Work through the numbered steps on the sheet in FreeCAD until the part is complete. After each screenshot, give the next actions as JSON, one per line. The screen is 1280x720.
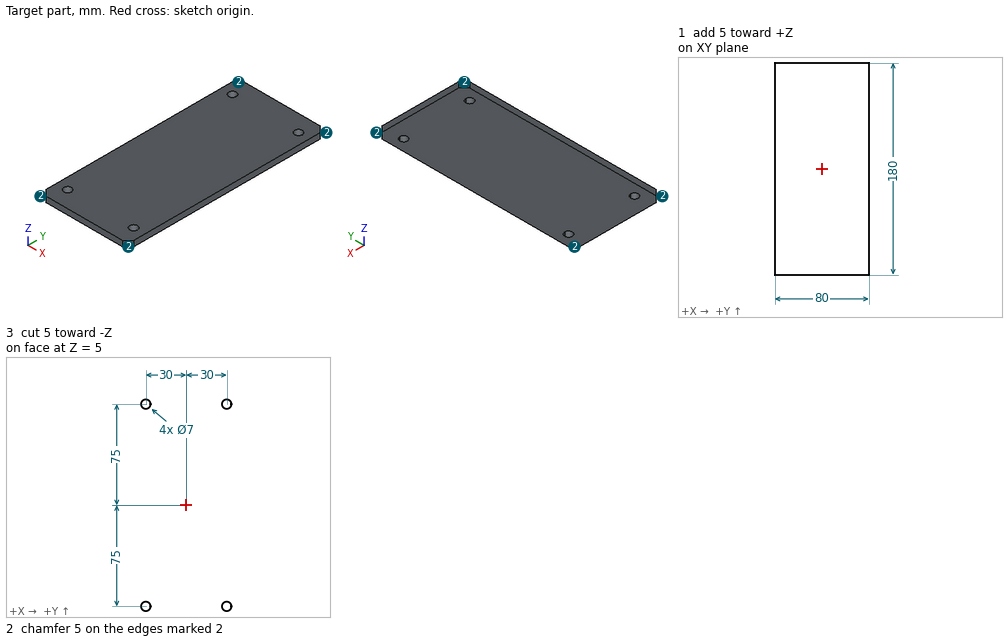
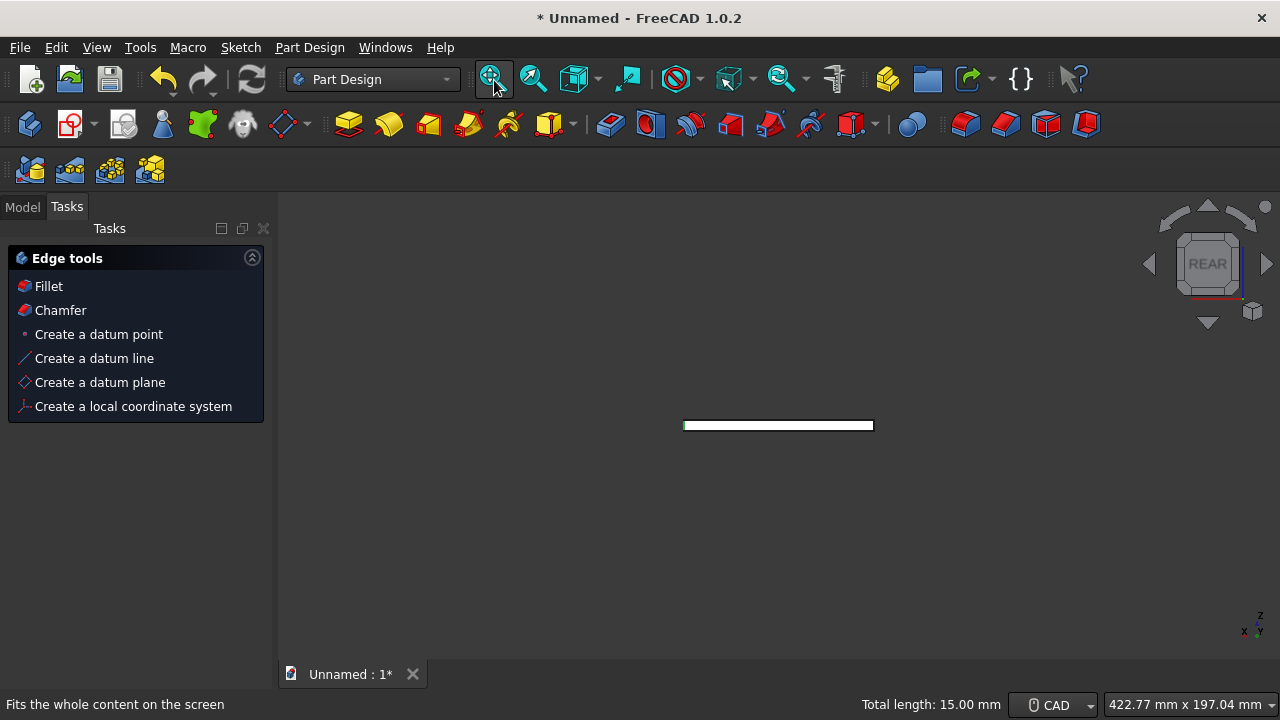
{"action": "scroll", "coordinate": [874, 425], "scroll_direction": "up", "scroll_amount": 7}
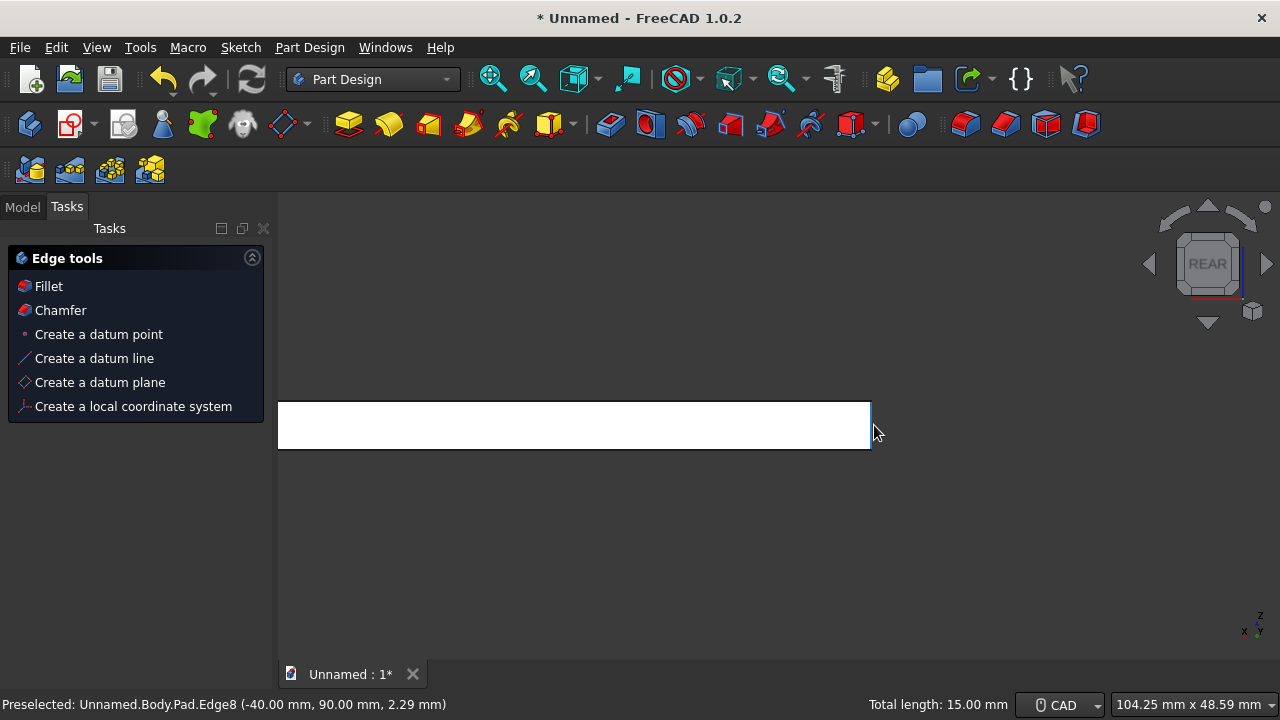
{"action": "left_click", "coordinate": [871, 425], "text": "ctrl"}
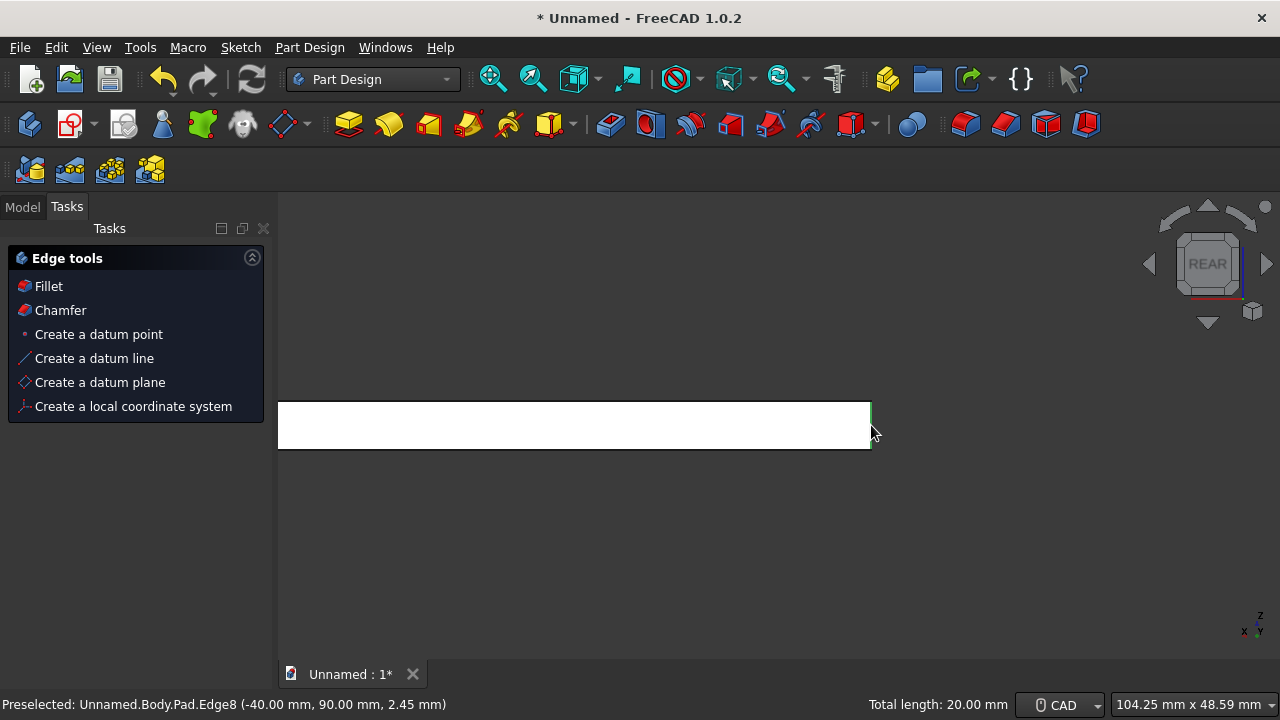
{"action": "left_click", "coordinate": [1006, 124]}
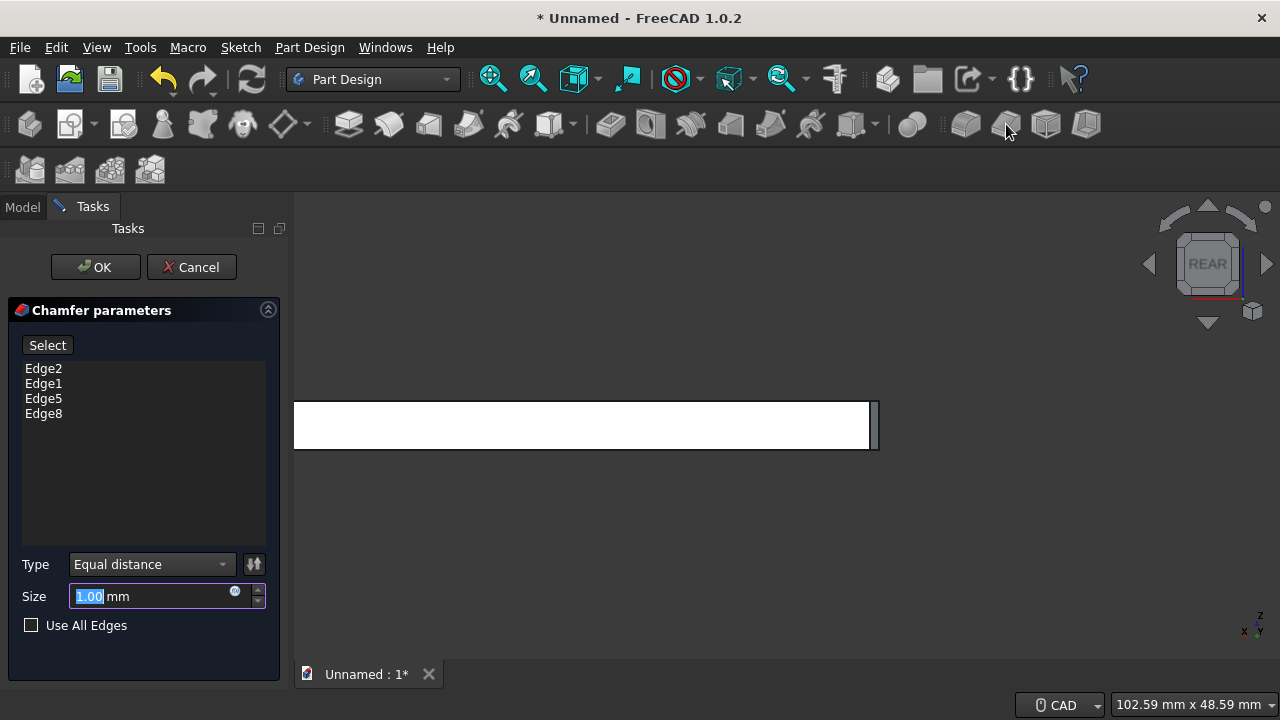
{"action": "type", "text": "5"}
{"action": "key", "text": "Tab"}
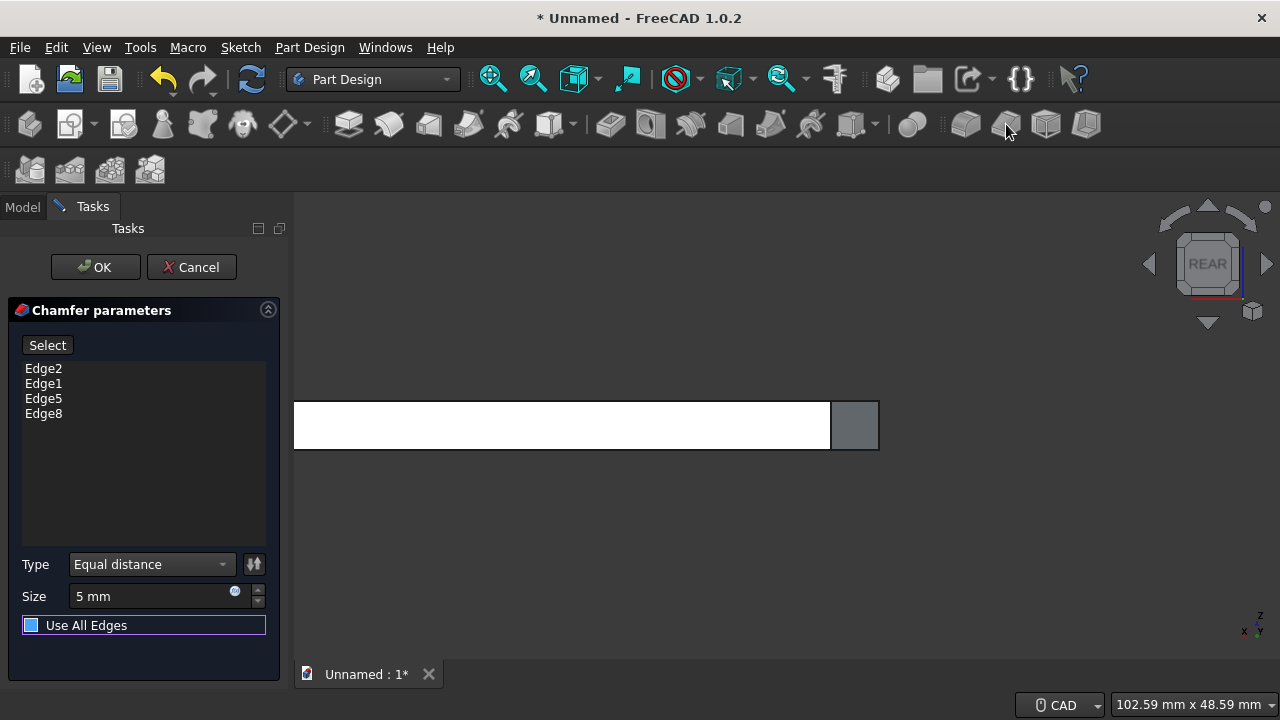
{"action": "left_click", "coordinate": [96, 267]}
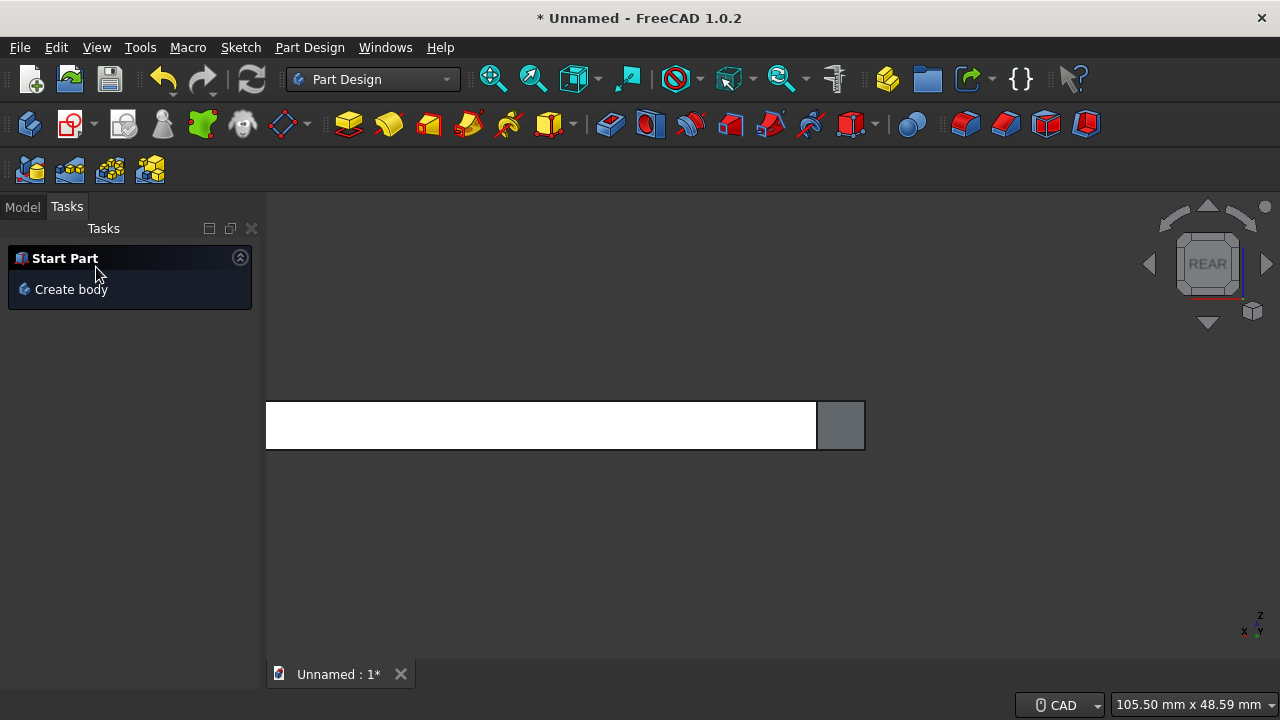
{"action": "left_click", "coordinate": [494, 80]}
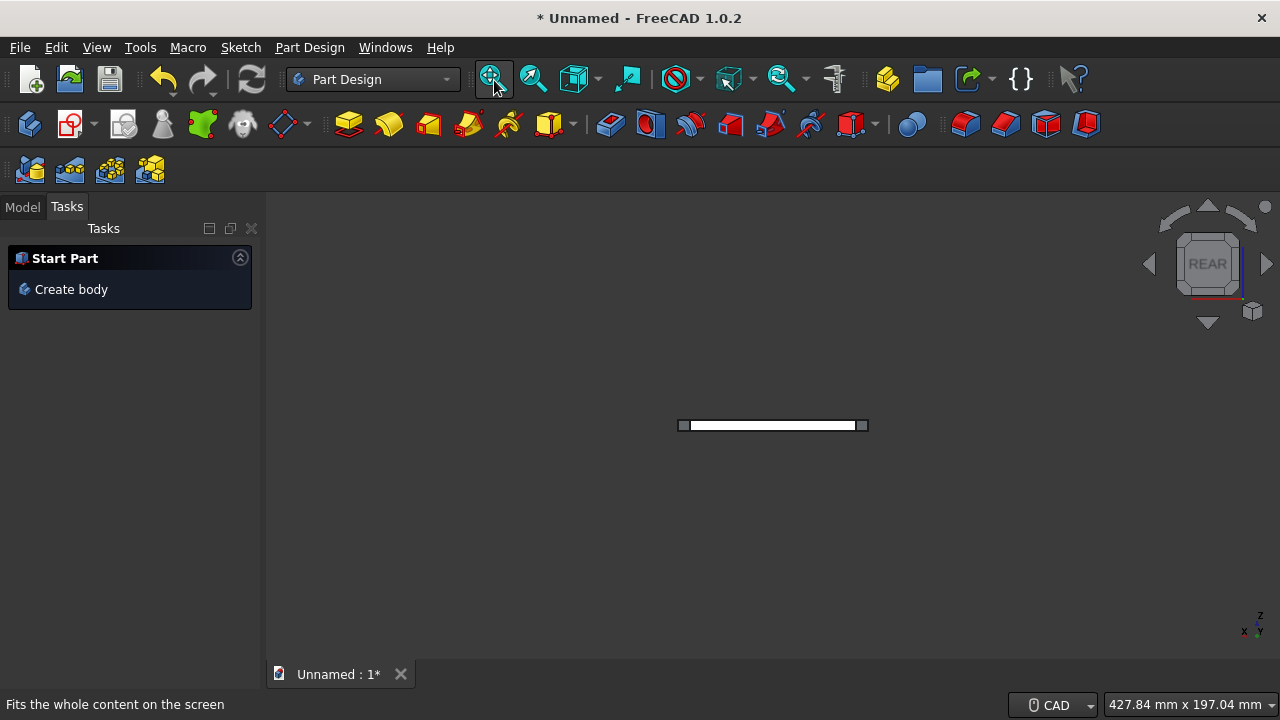
{"action": "key", "text": "0"}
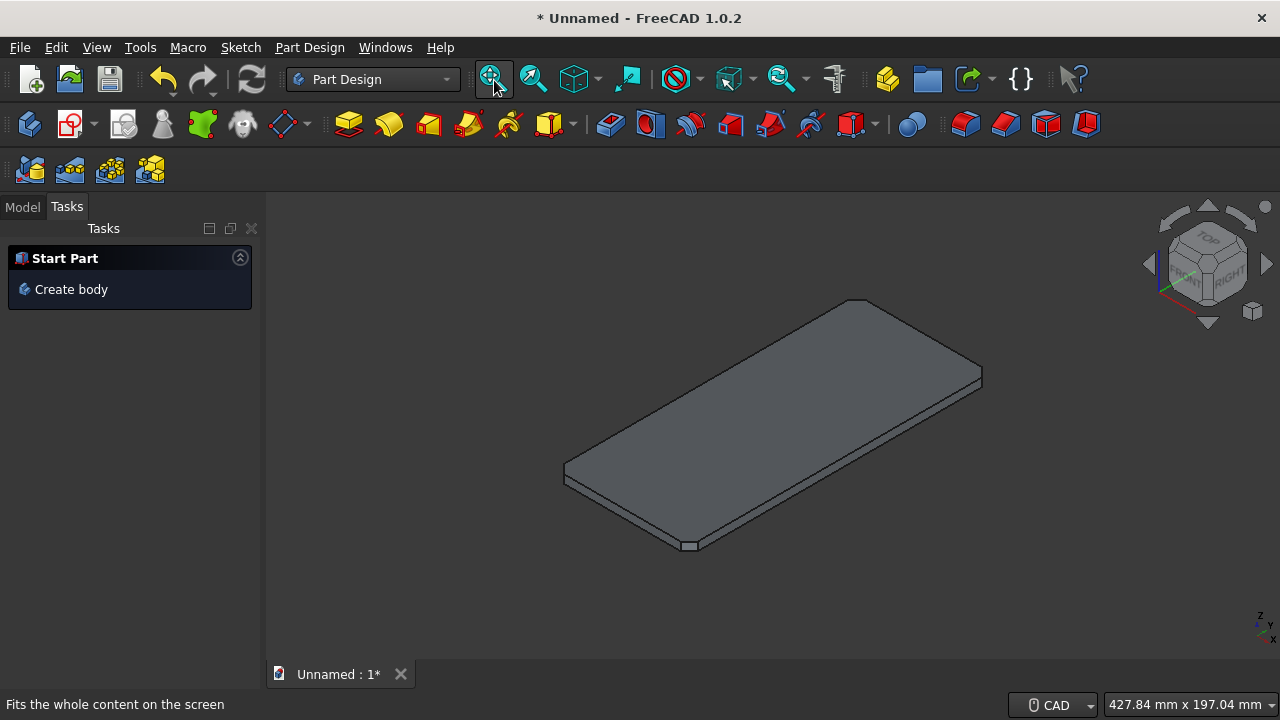
{"action": "left_click", "coordinate": [816, 395]}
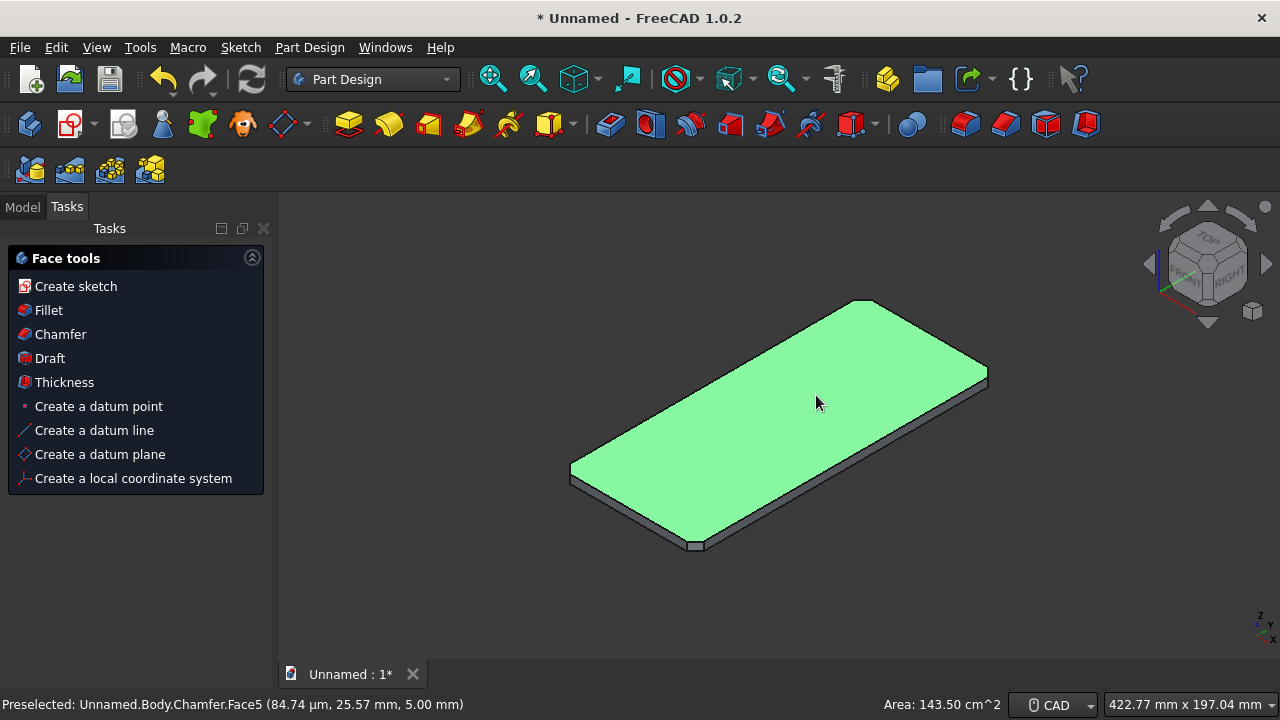
{"action": "left_click", "coordinate": [70, 124]}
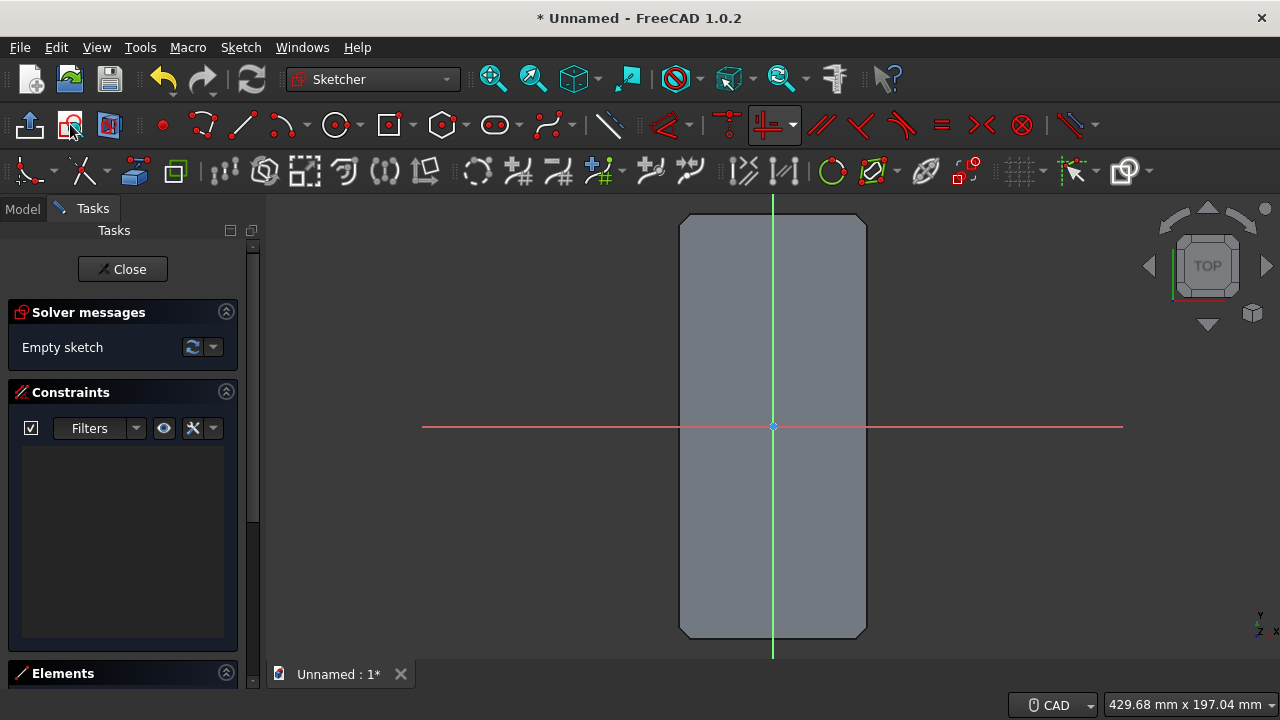
{"action": "scroll", "coordinate": [395, 427], "scroll_direction": "down", "scroll_amount": 1}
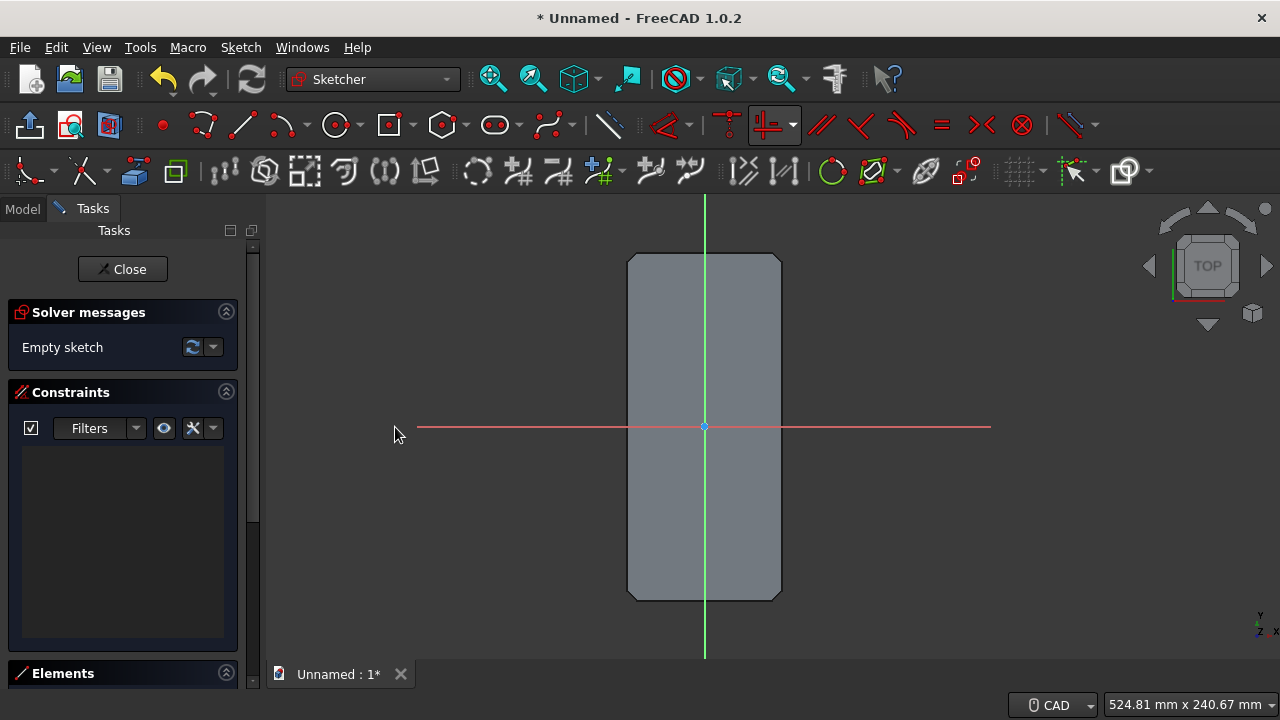
{"action": "left_click", "coordinate": [336, 126]}